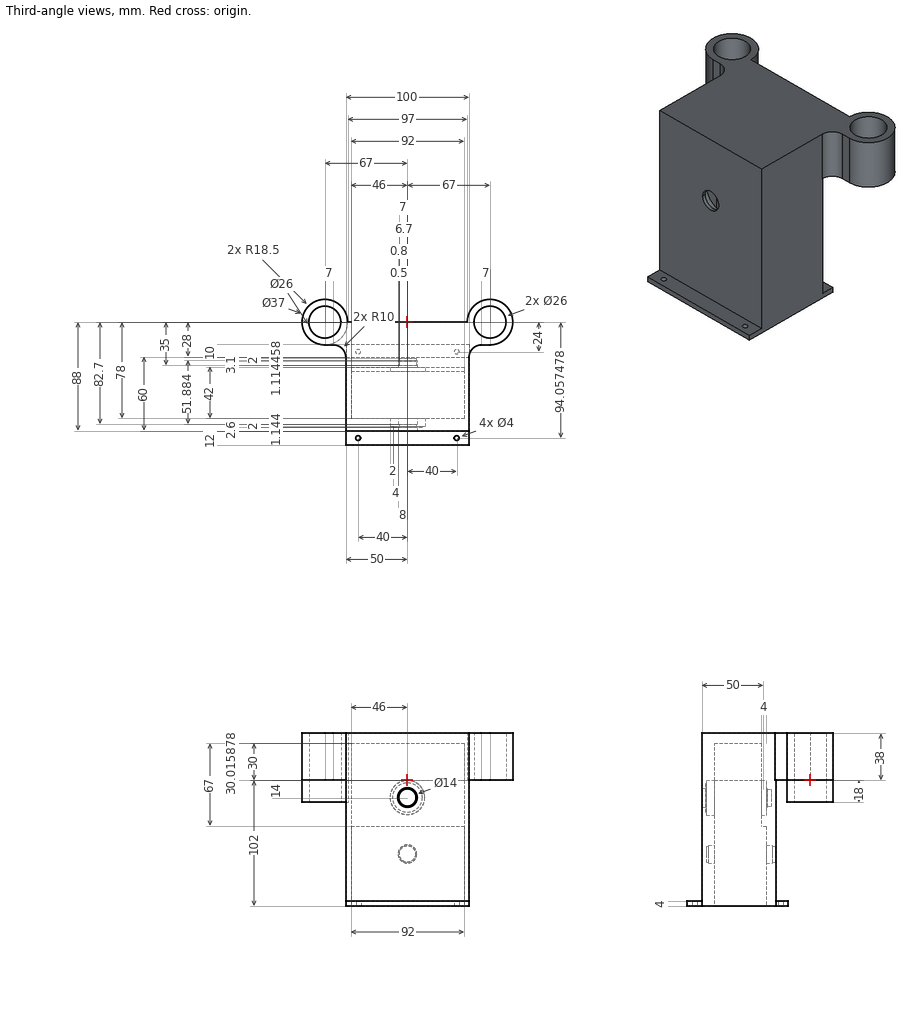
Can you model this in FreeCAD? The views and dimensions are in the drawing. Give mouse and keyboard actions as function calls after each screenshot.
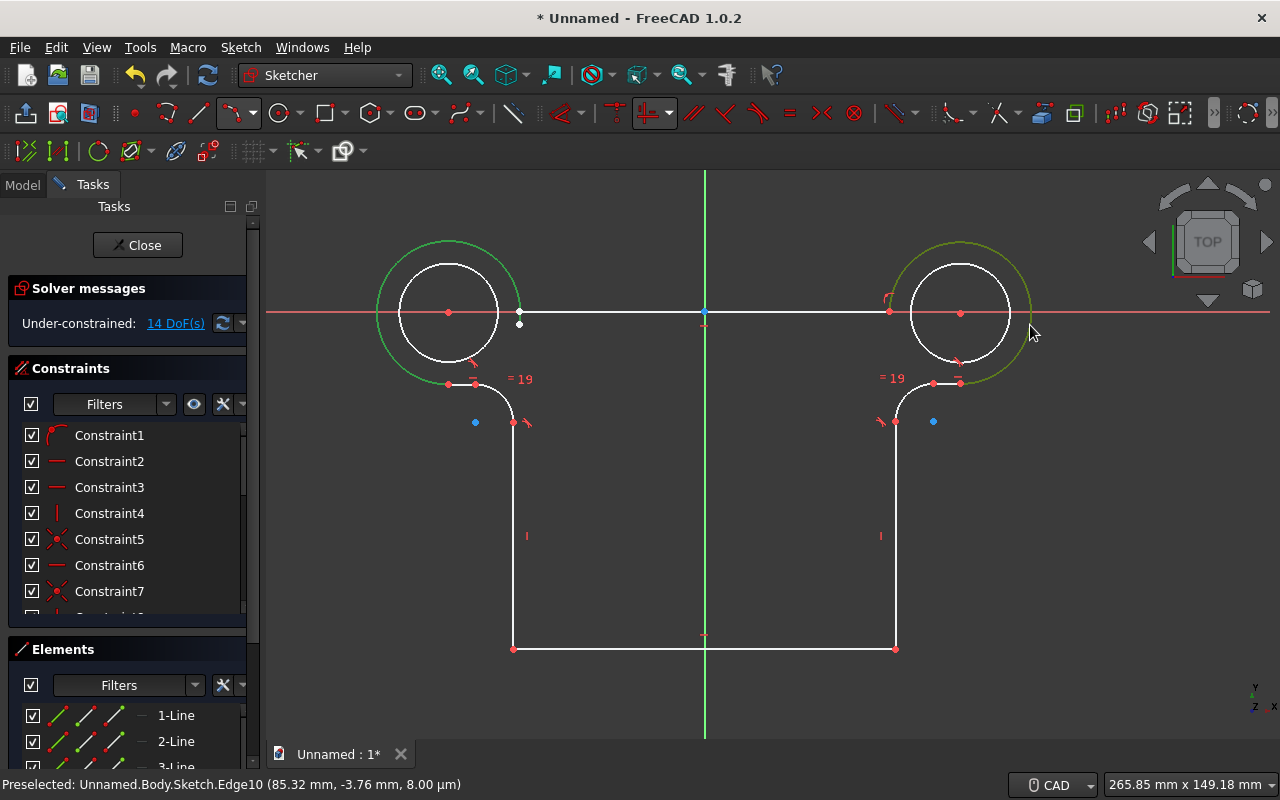
key(e)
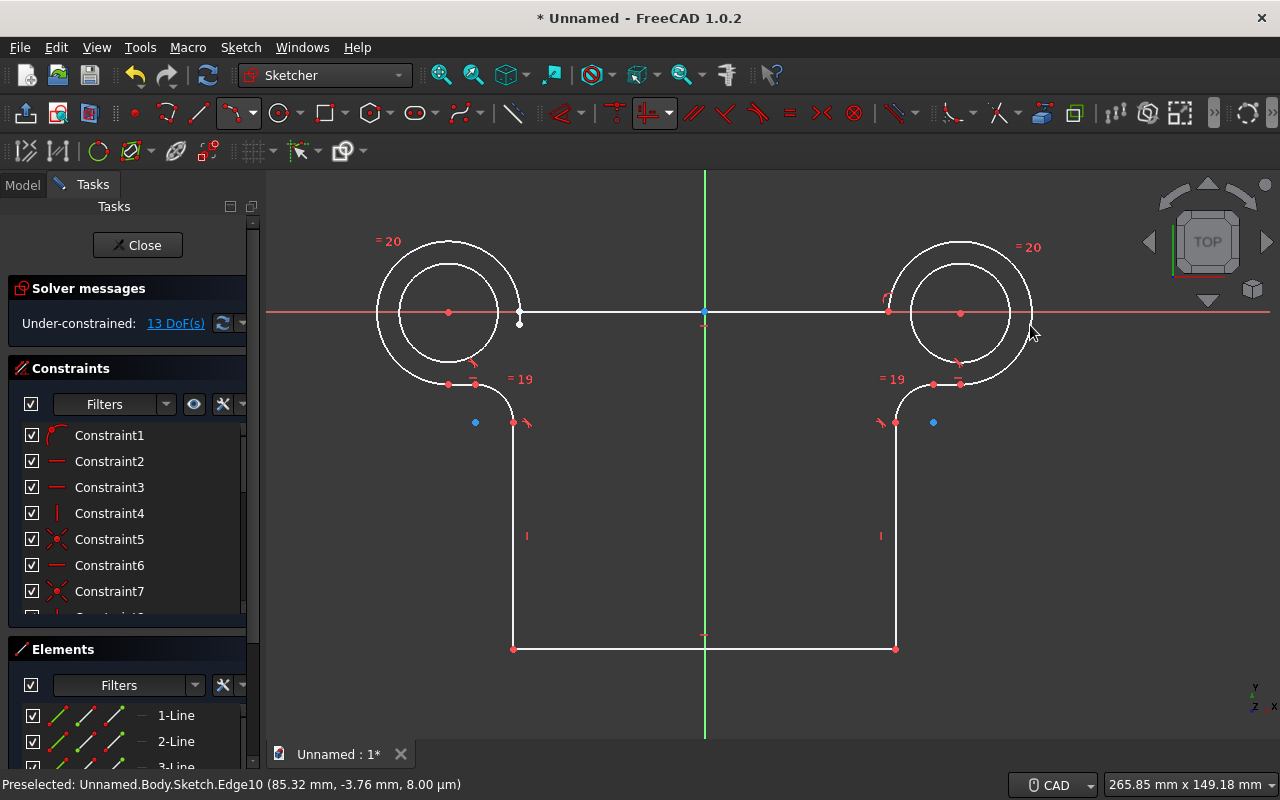
click(995, 278)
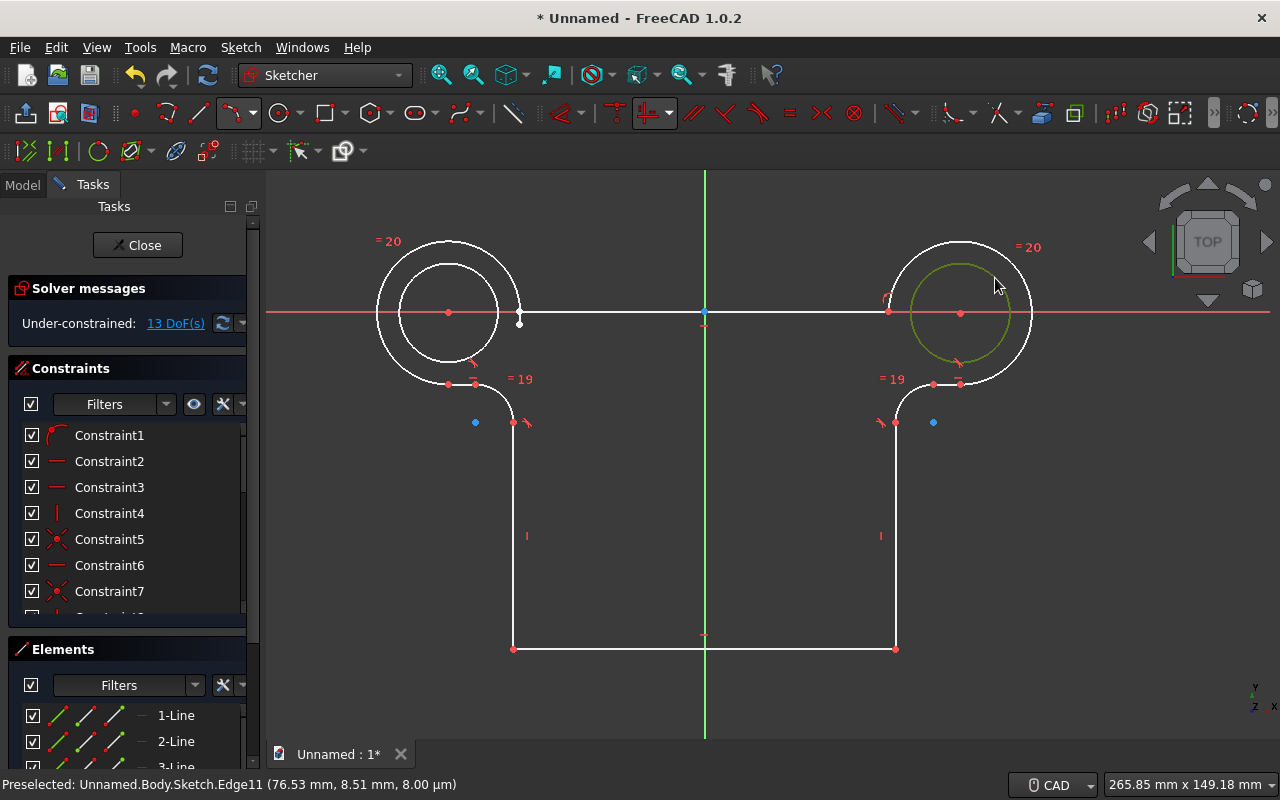
click(483, 278)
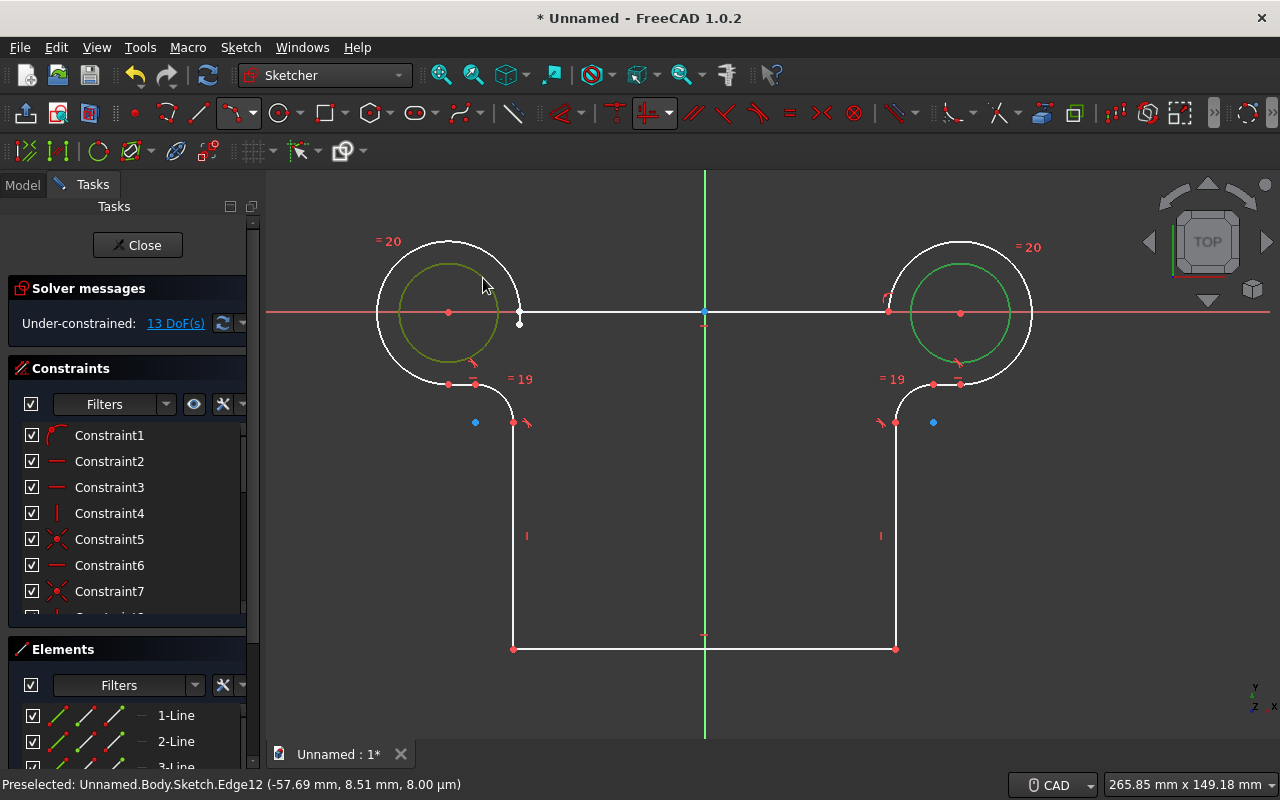
click(790, 114)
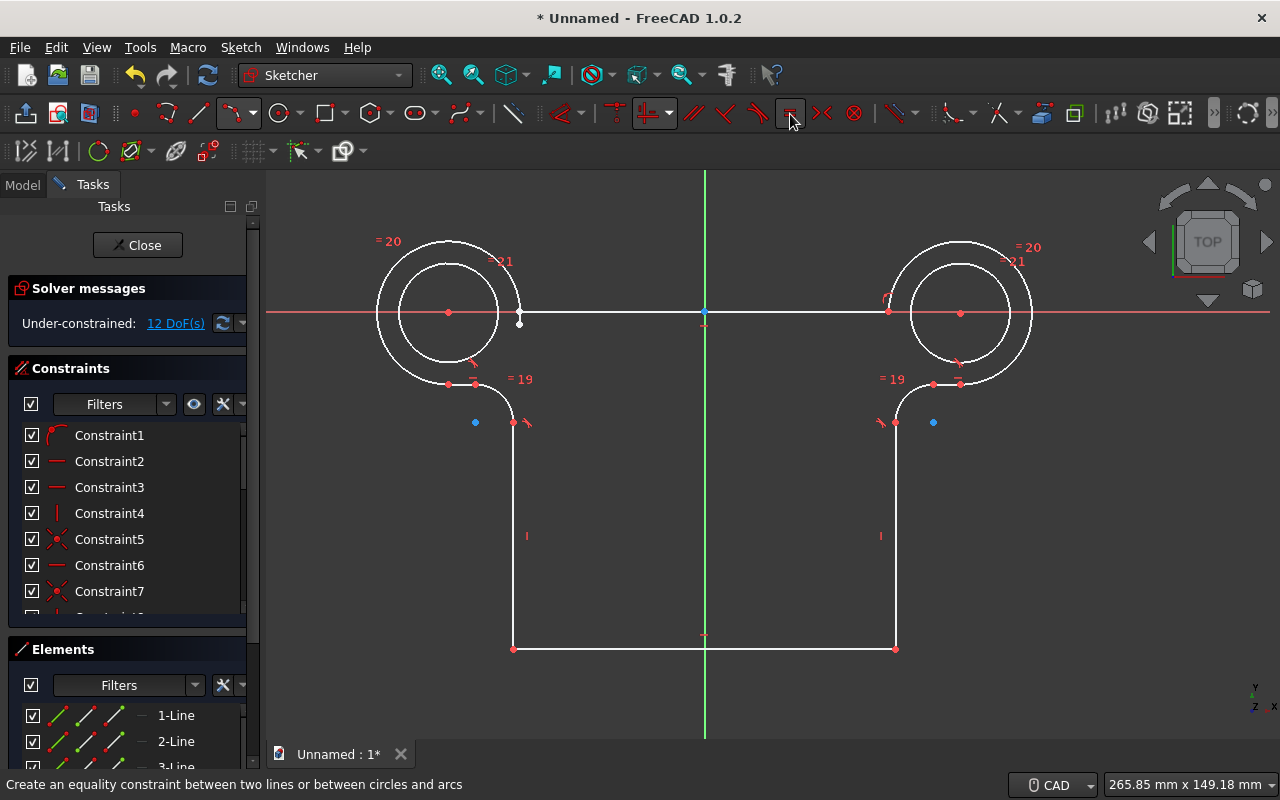
click(449, 313)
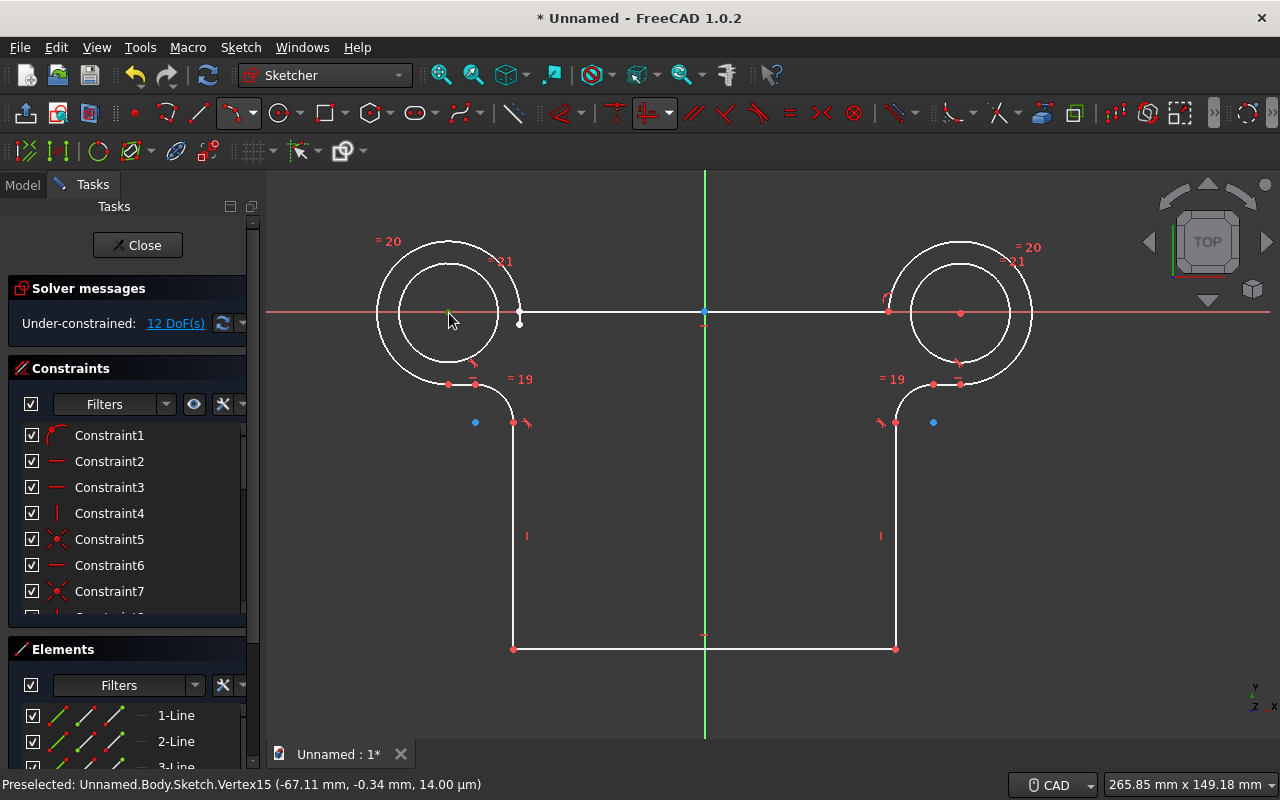
click(939, 312)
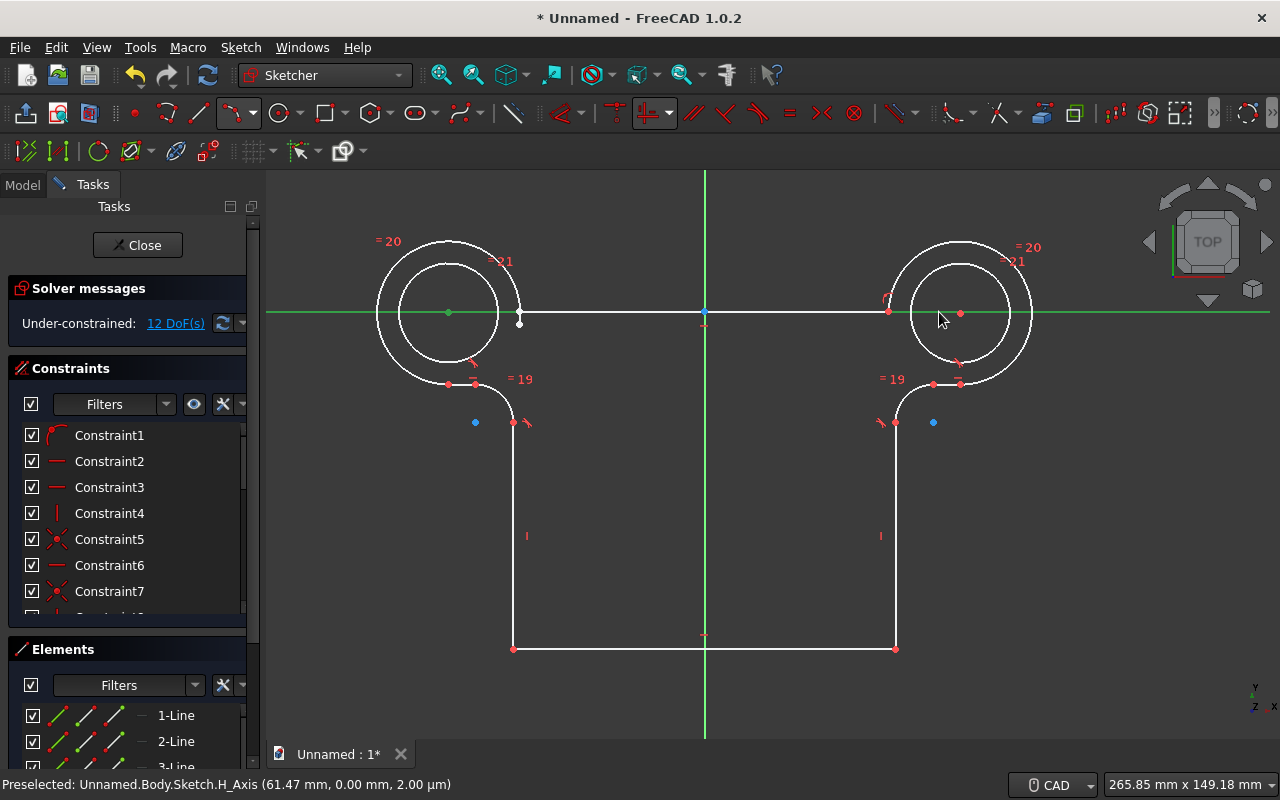
key(c)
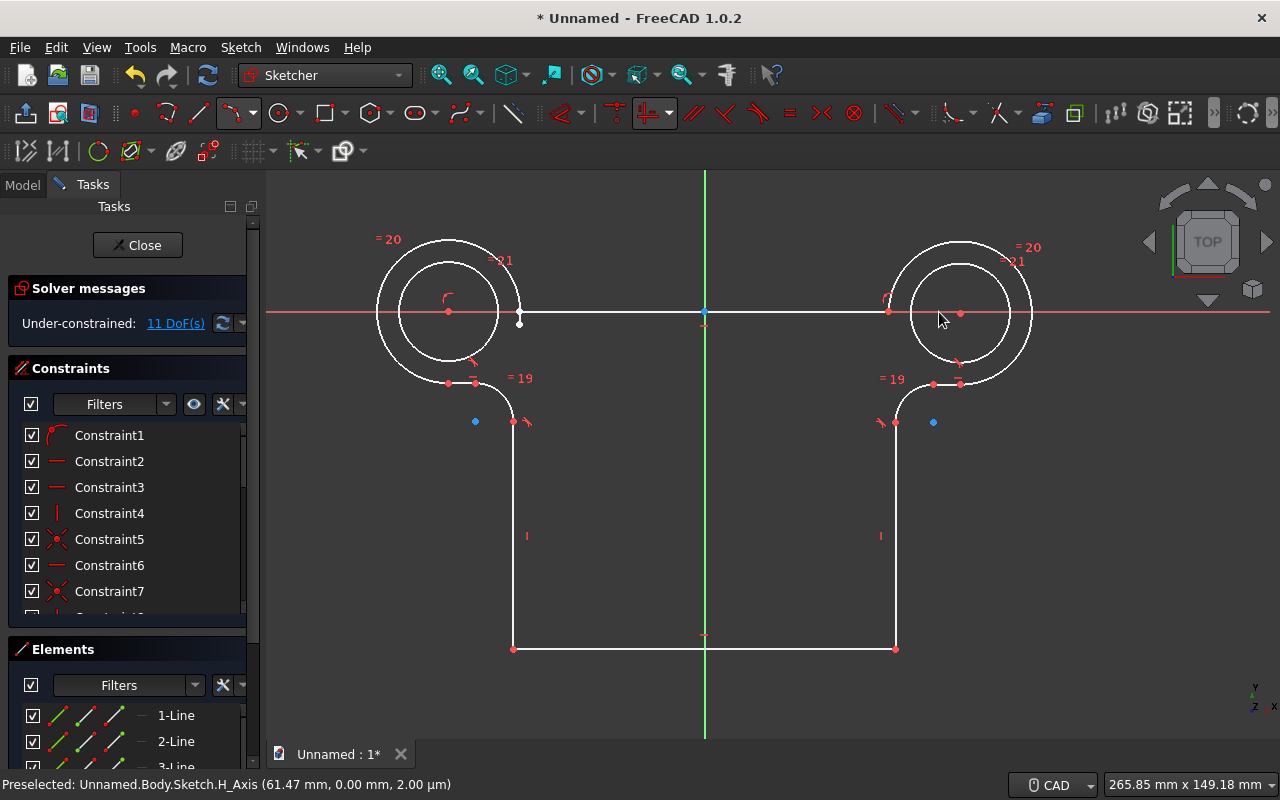
click(960, 313)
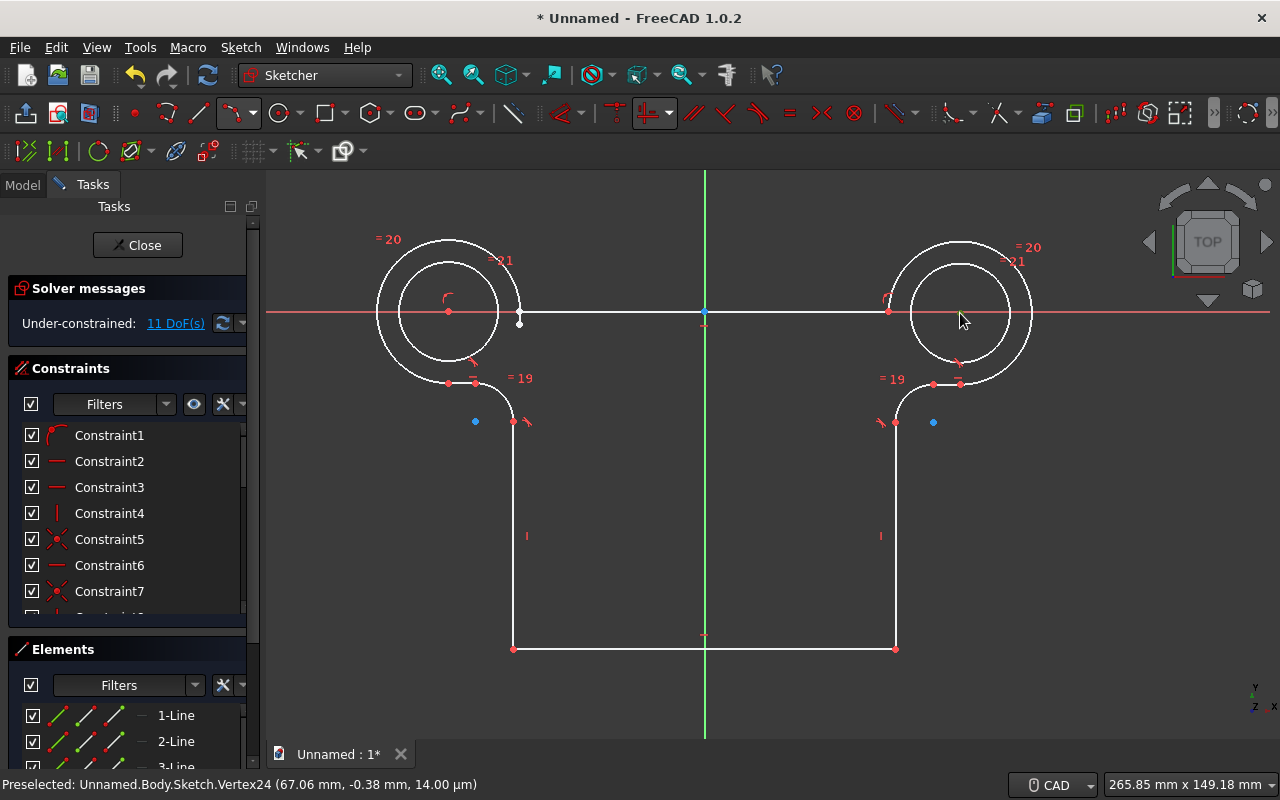
click(939, 312)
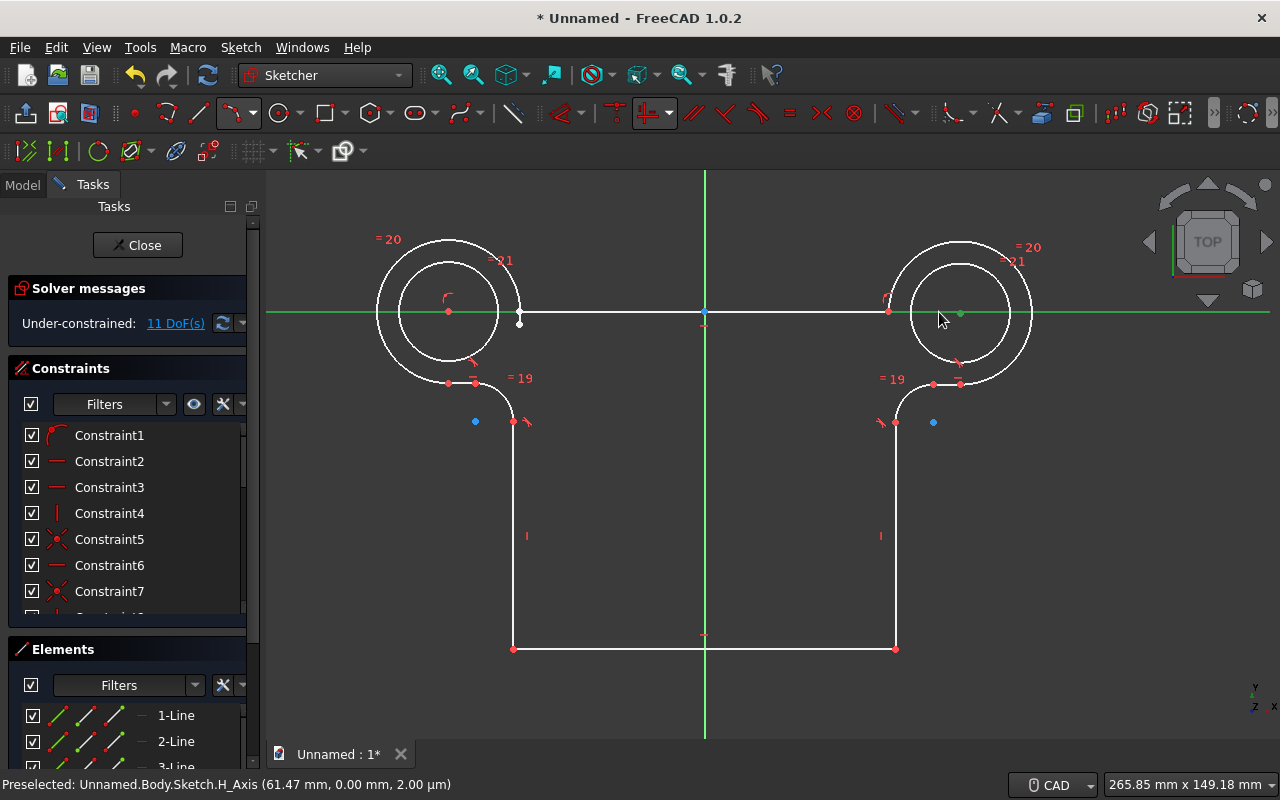
key(c)